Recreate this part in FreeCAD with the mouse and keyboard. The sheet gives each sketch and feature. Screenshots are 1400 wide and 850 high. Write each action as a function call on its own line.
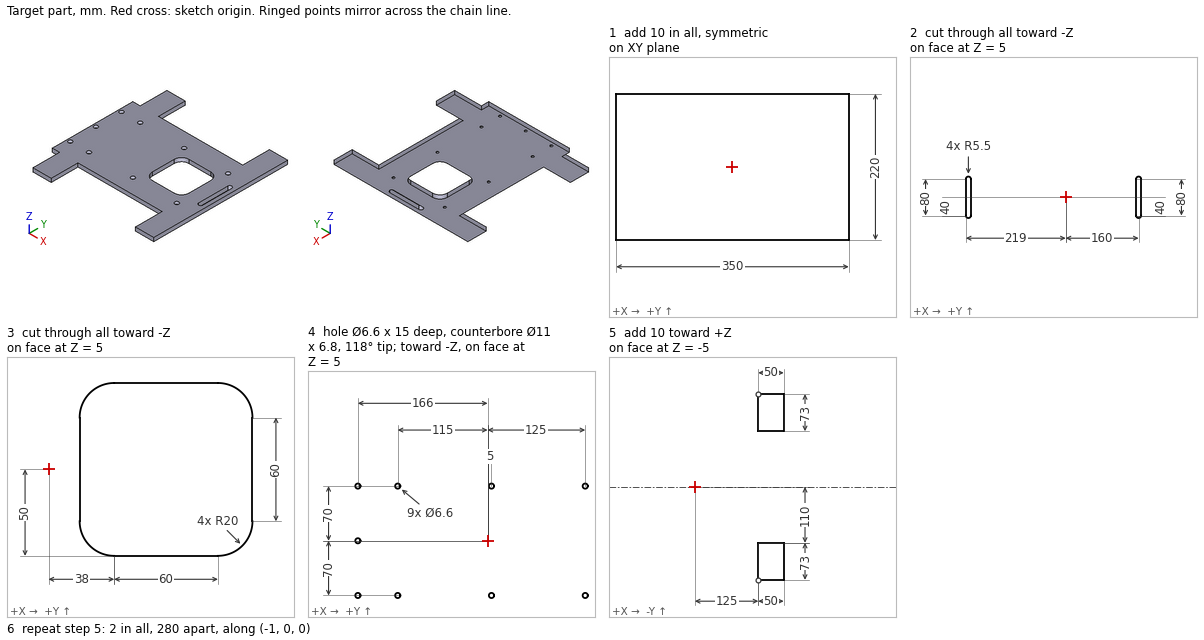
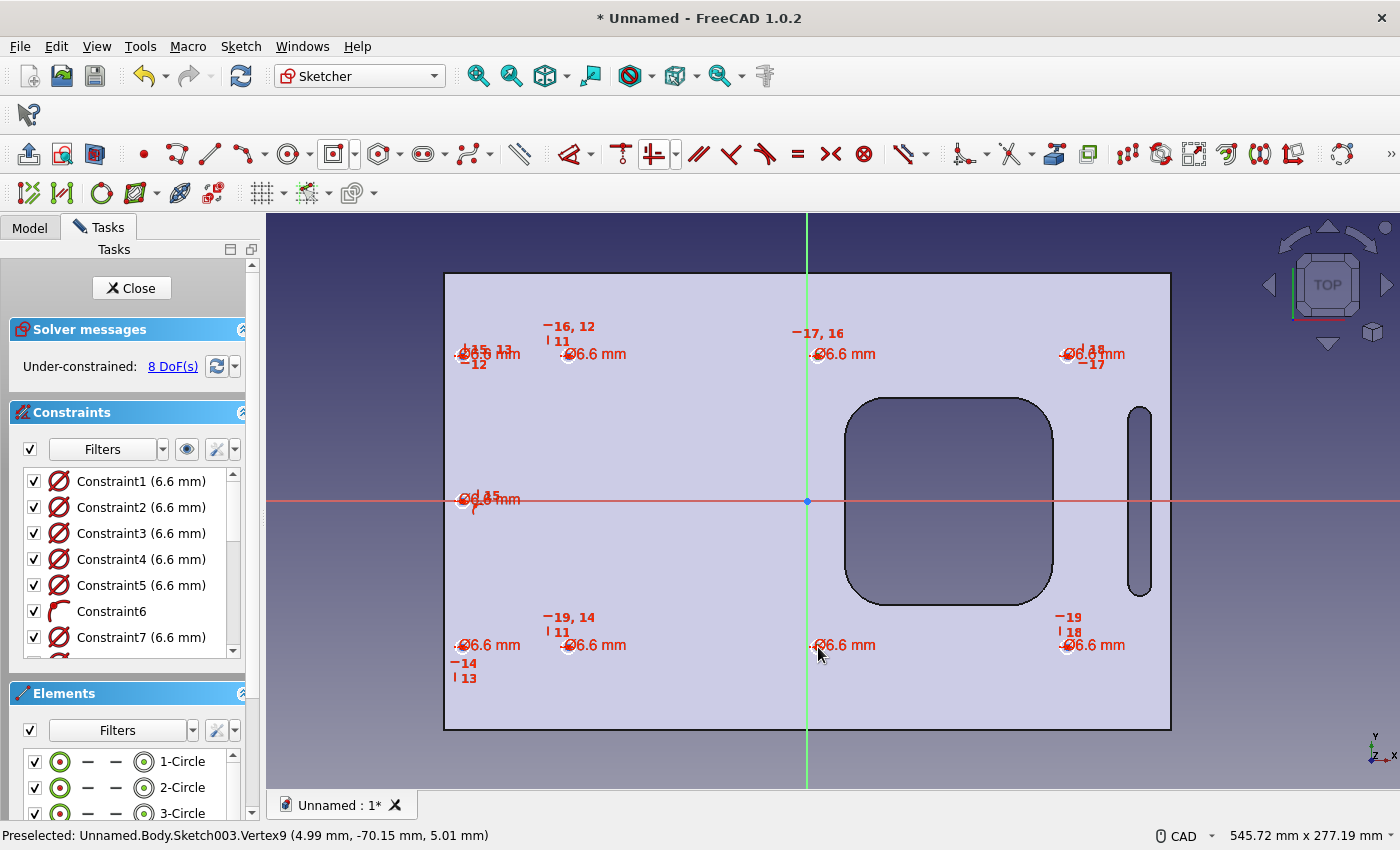
click(676, 154)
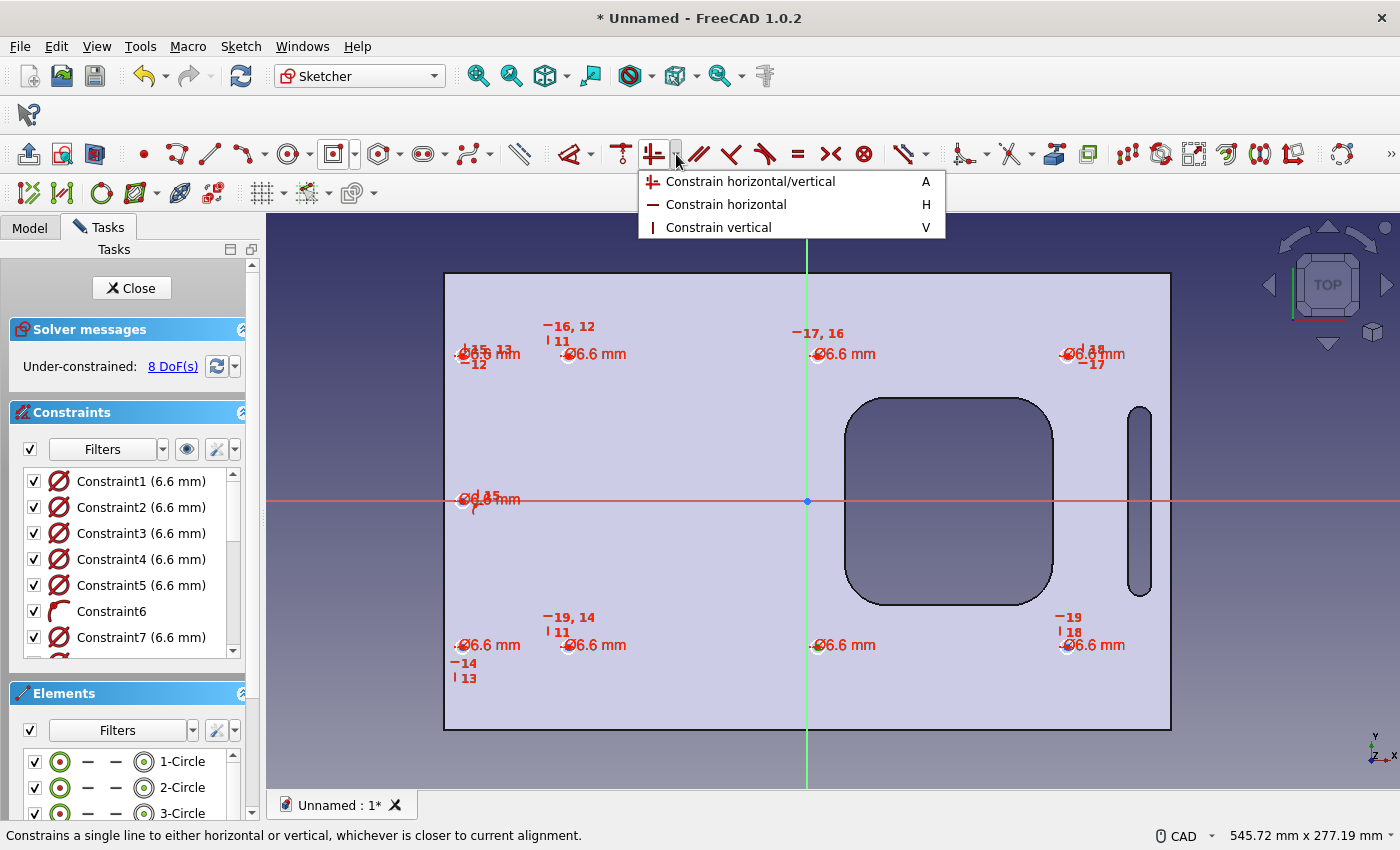
click(792, 228)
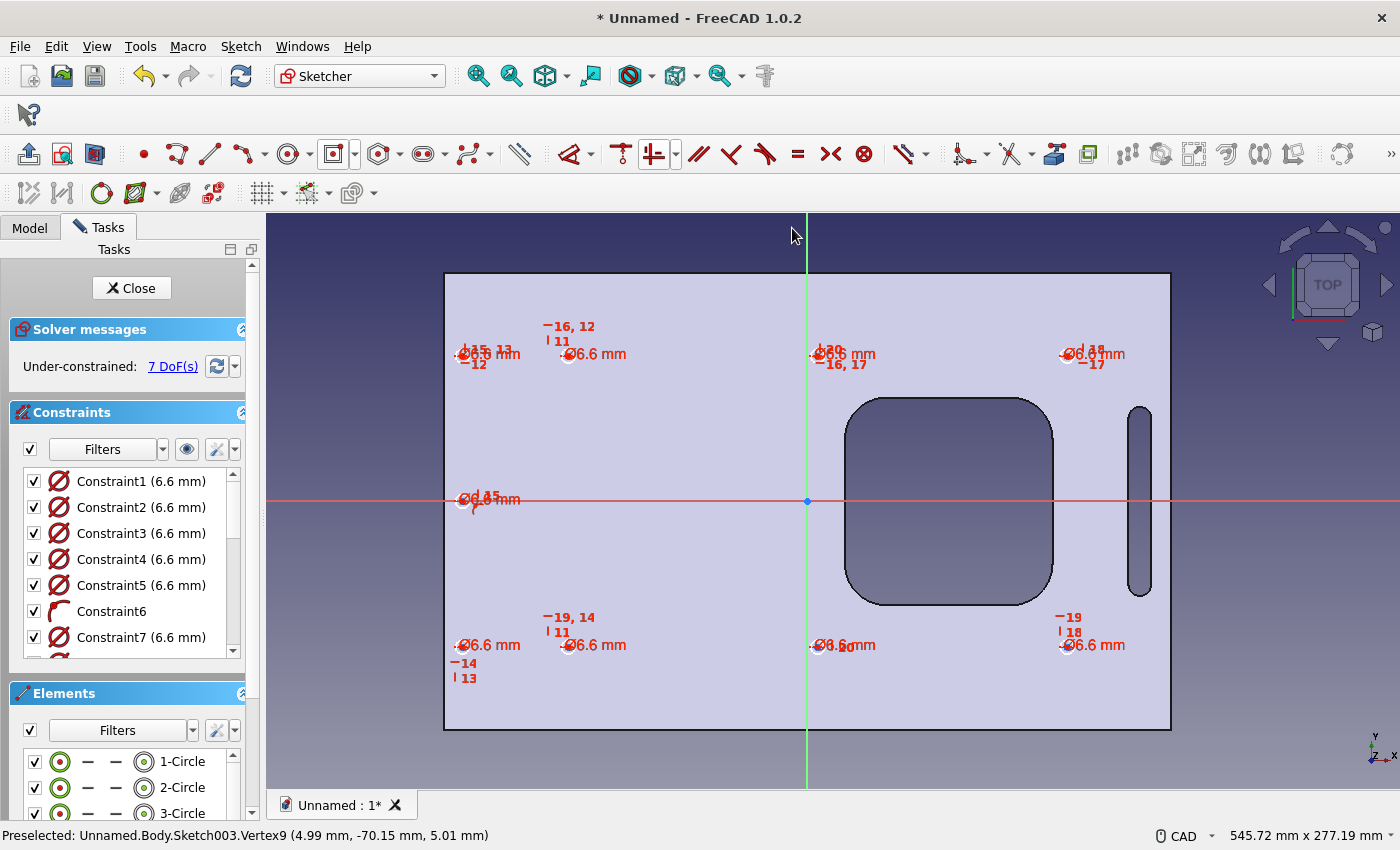
click(568, 647)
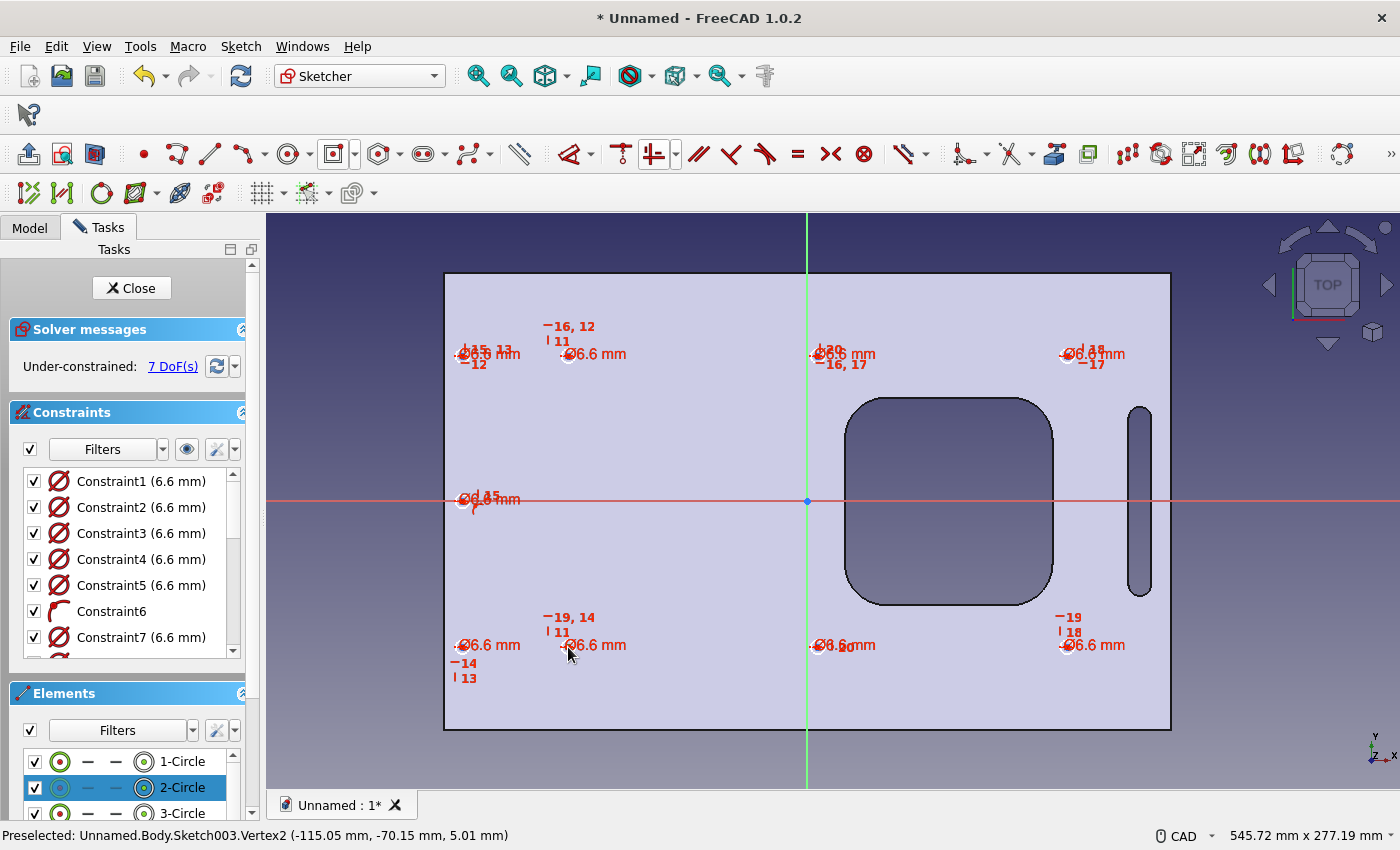
click(818, 647)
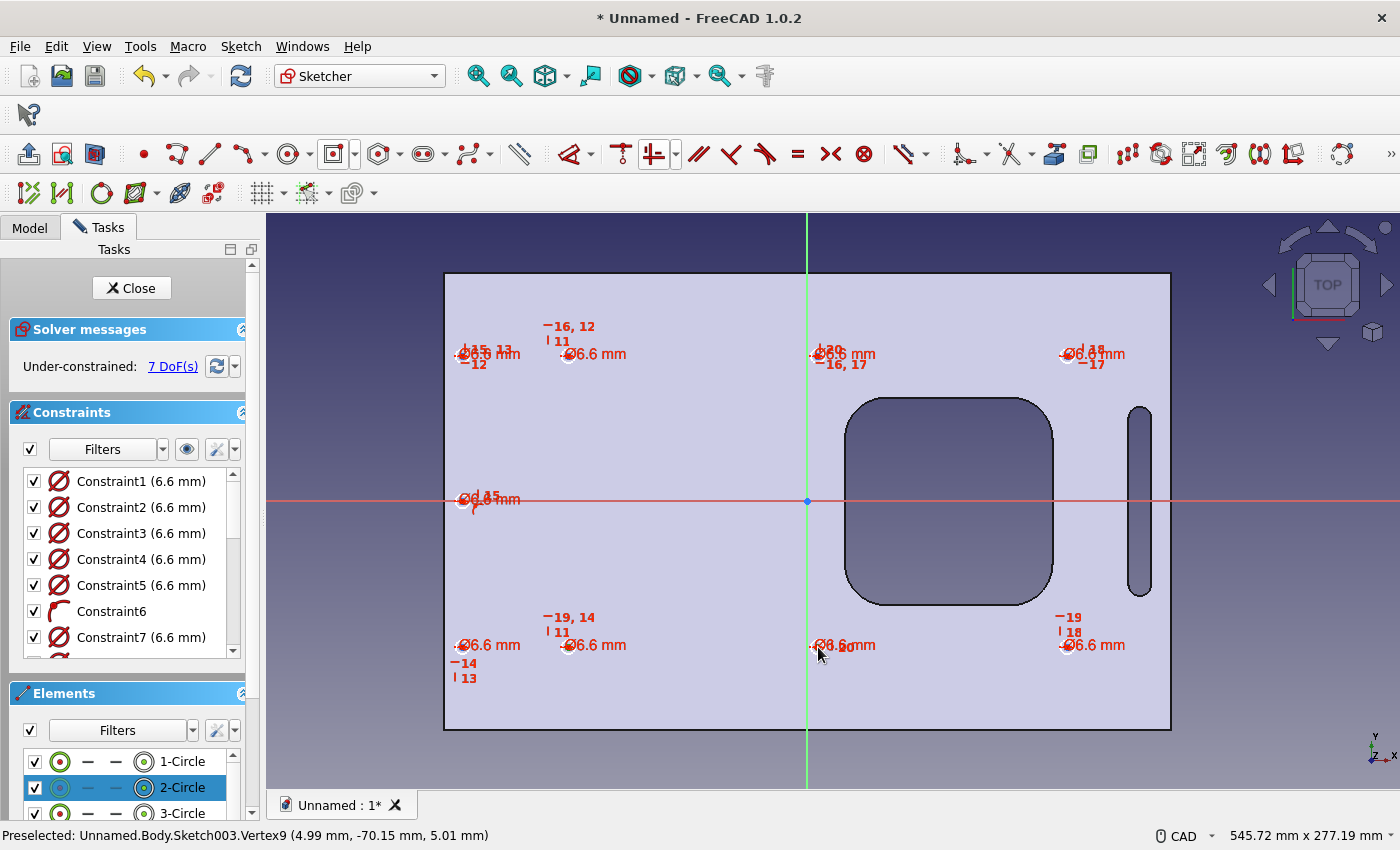
click(676, 154)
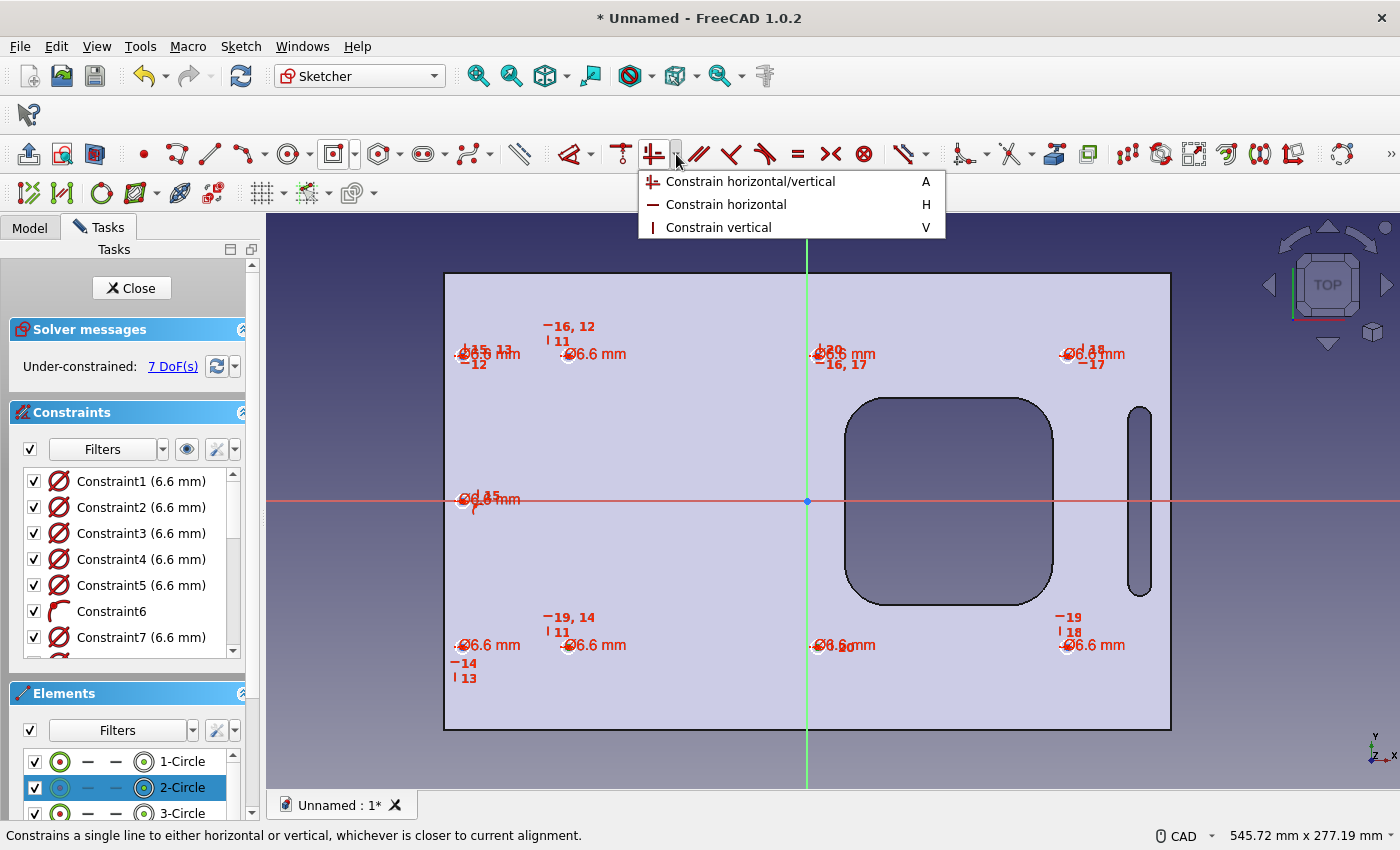
click(792, 204)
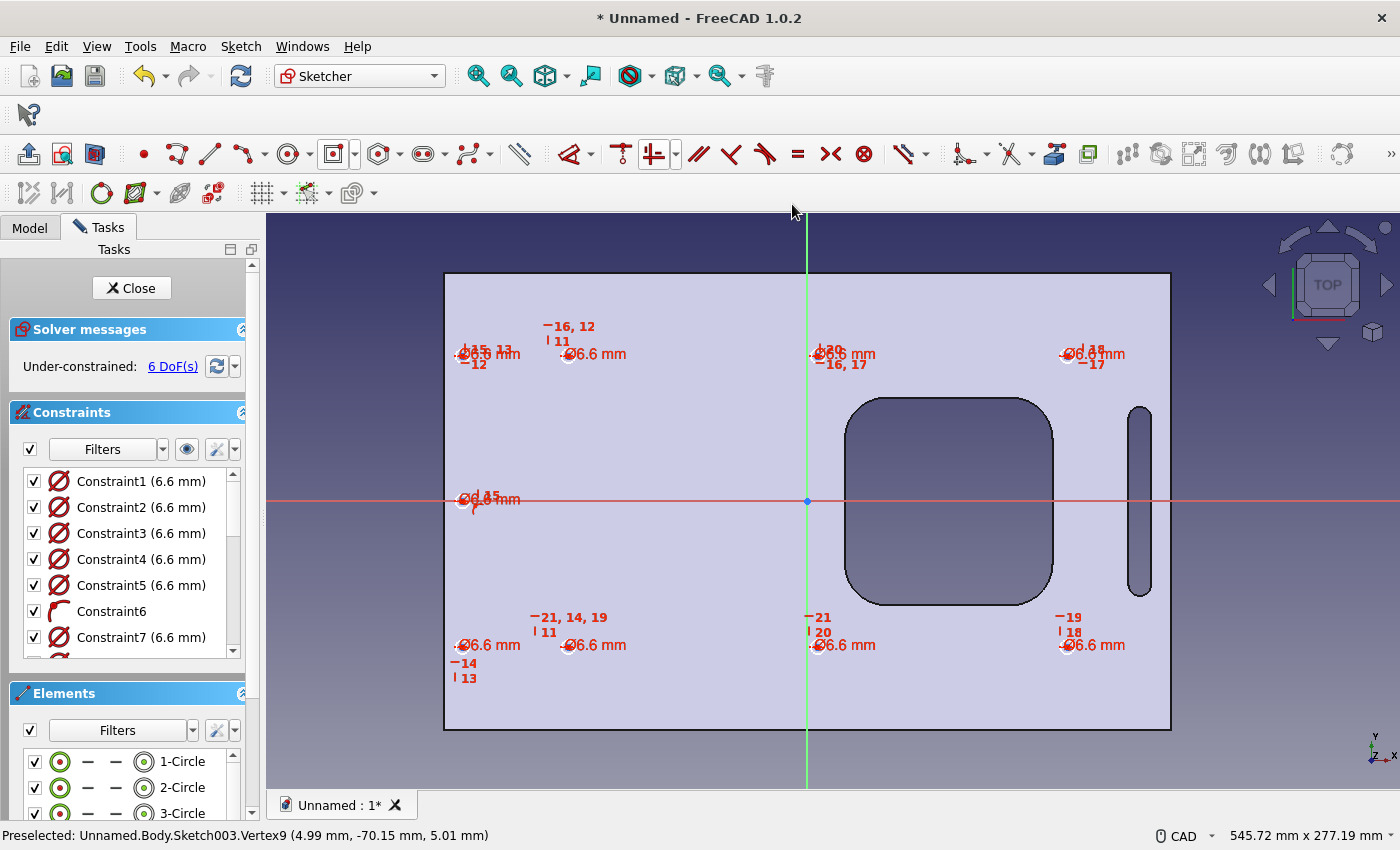
click(568, 154)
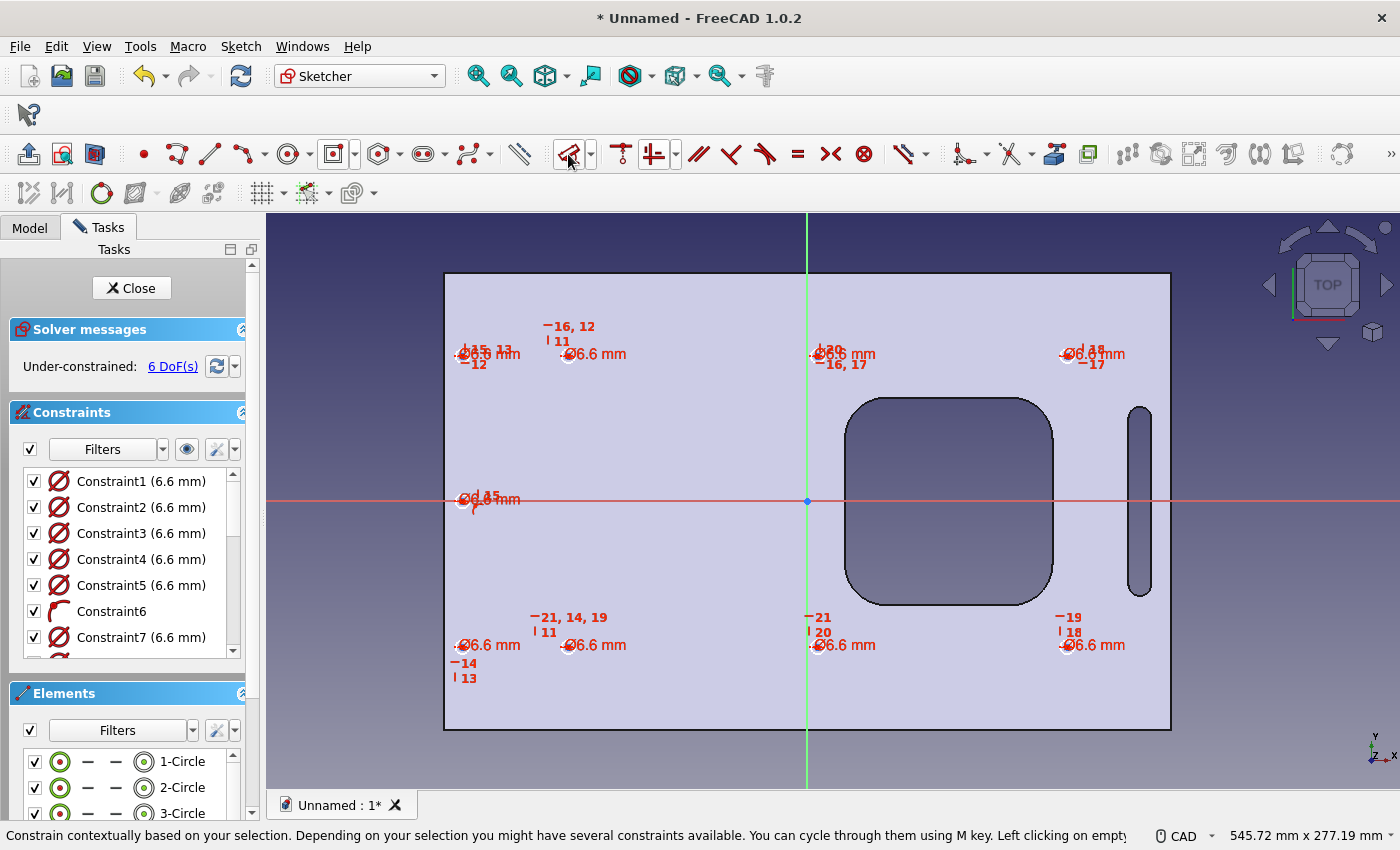
scroll(818, 356, up, 7)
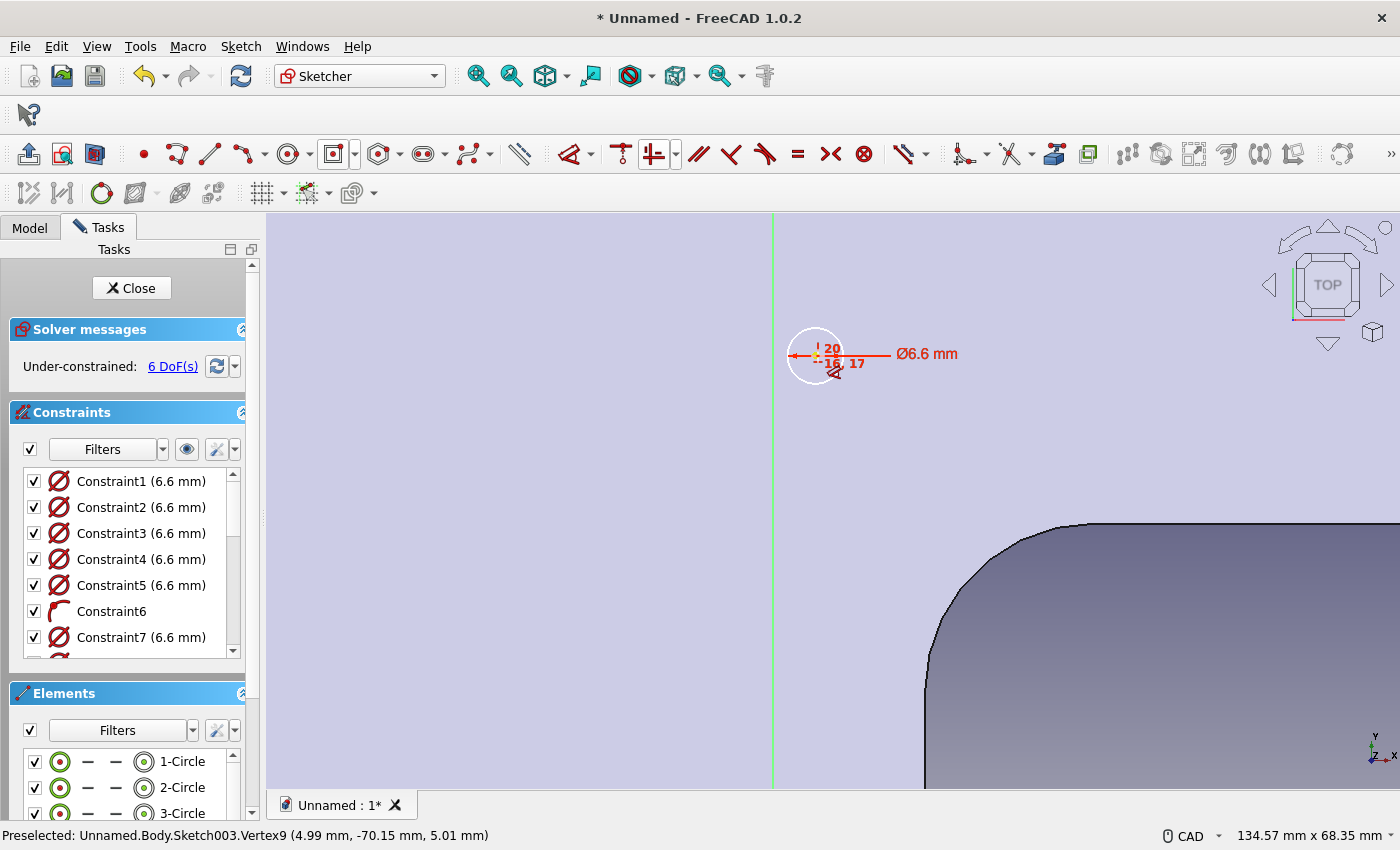
click(815, 356)
click(794, 298)